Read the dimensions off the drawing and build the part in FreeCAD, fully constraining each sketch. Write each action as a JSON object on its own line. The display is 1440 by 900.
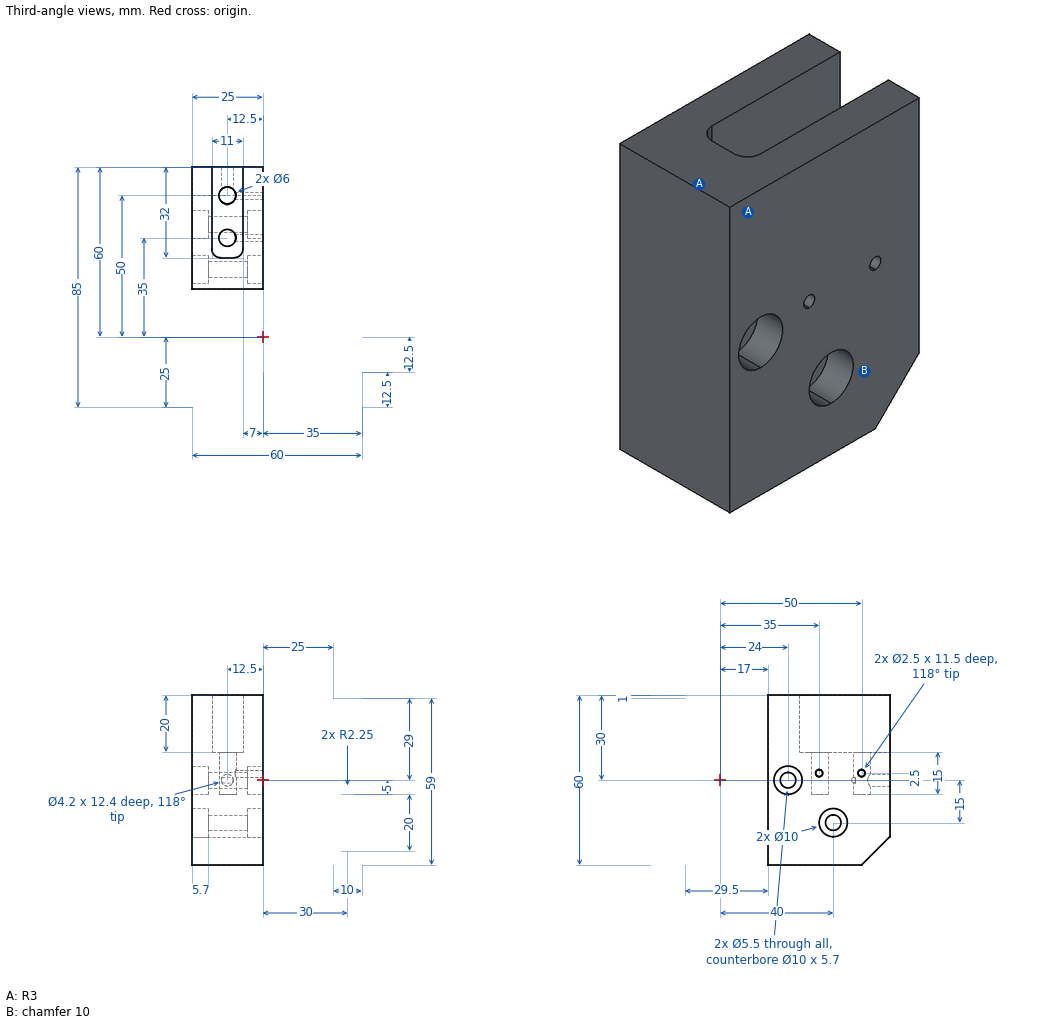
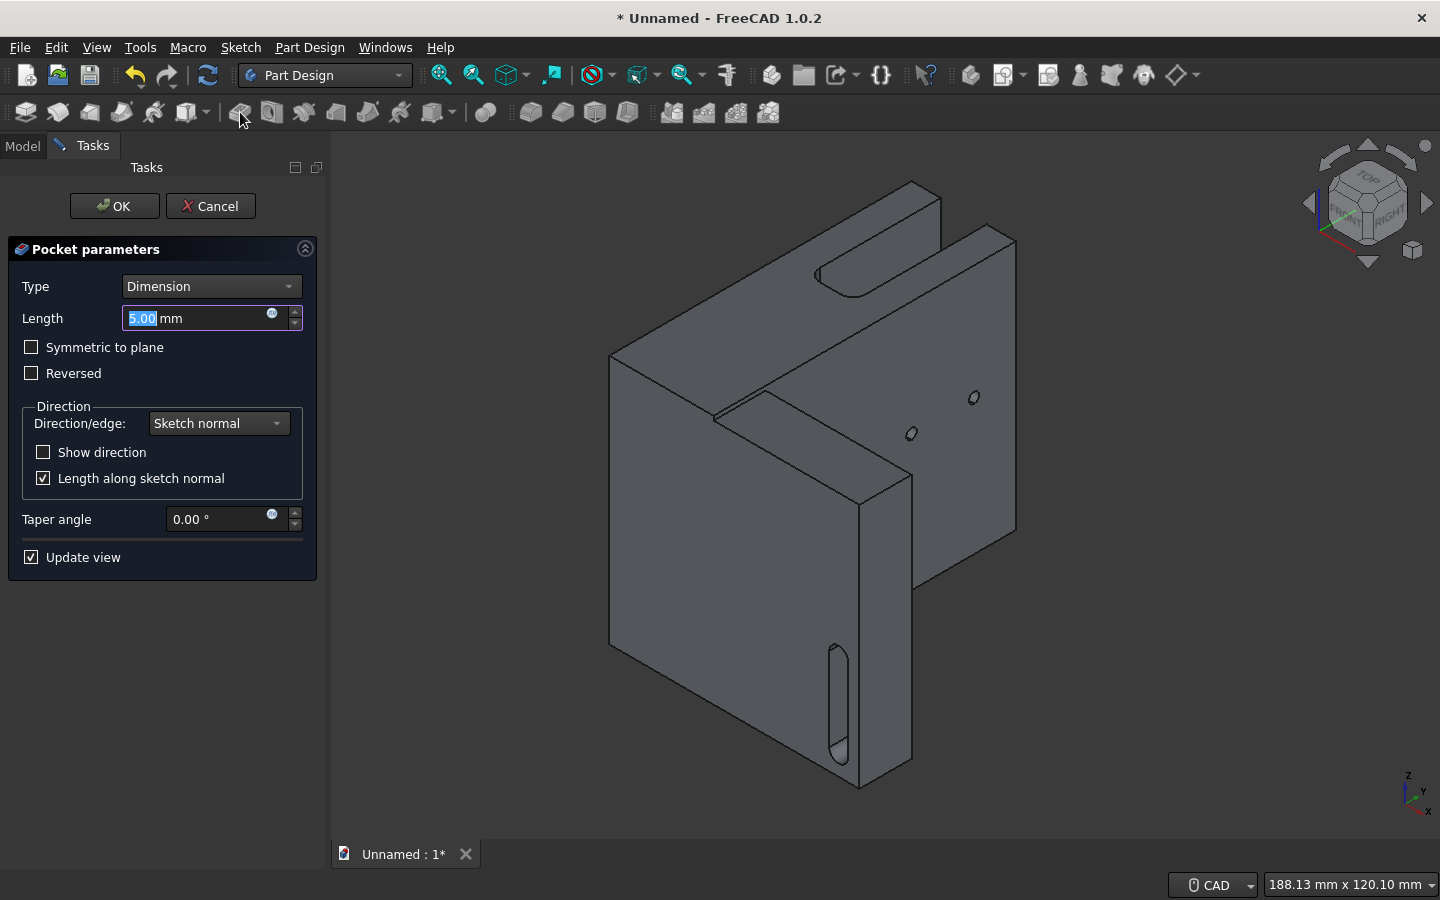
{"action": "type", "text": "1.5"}
{"action": "key", "text": "Tab"}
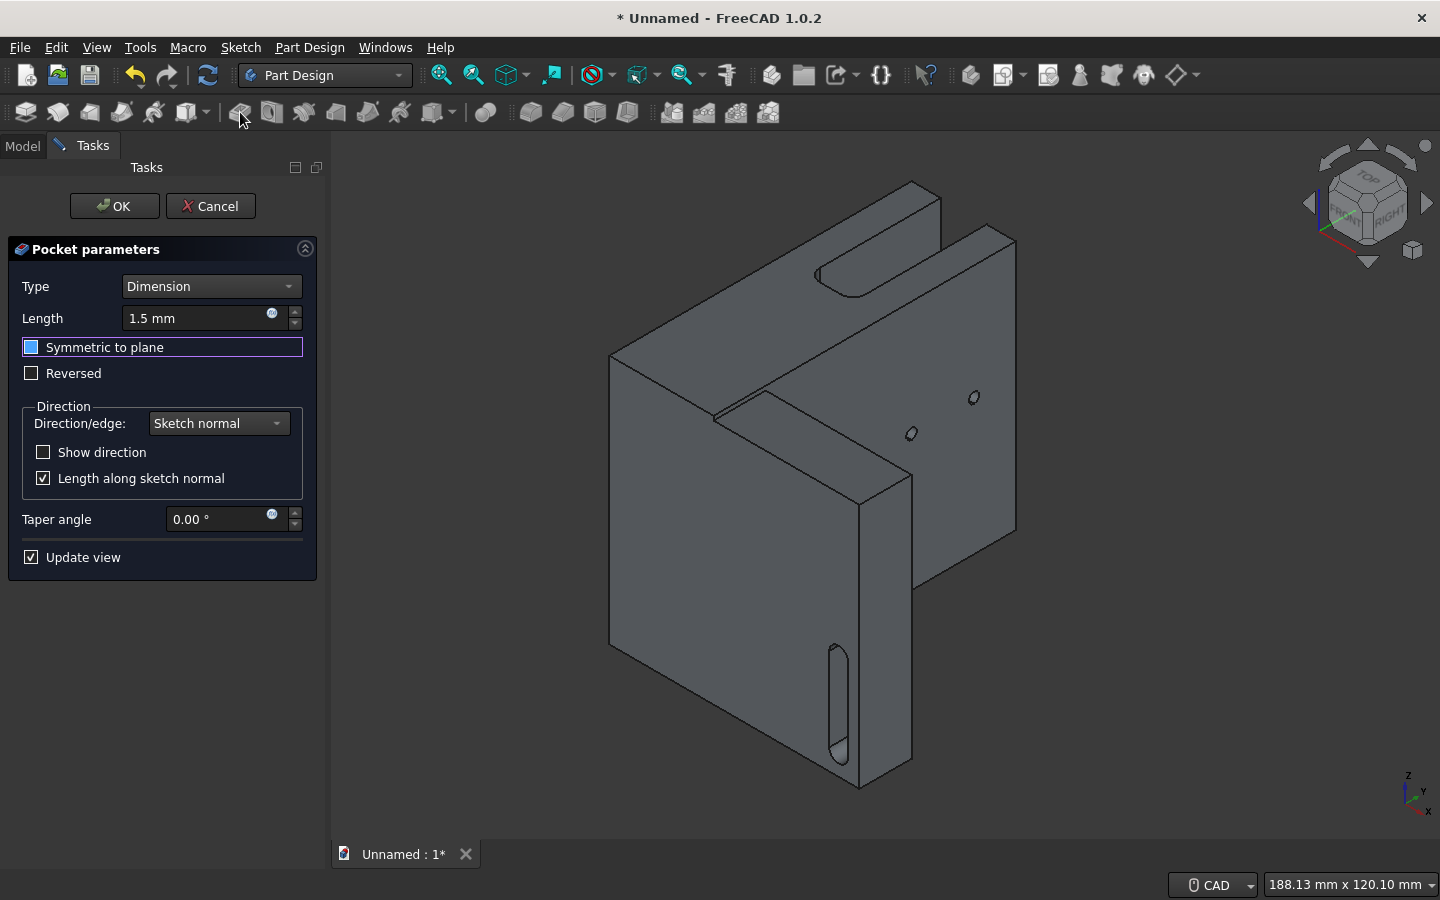
{"action": "left_click", "coordinate": [30, 373]}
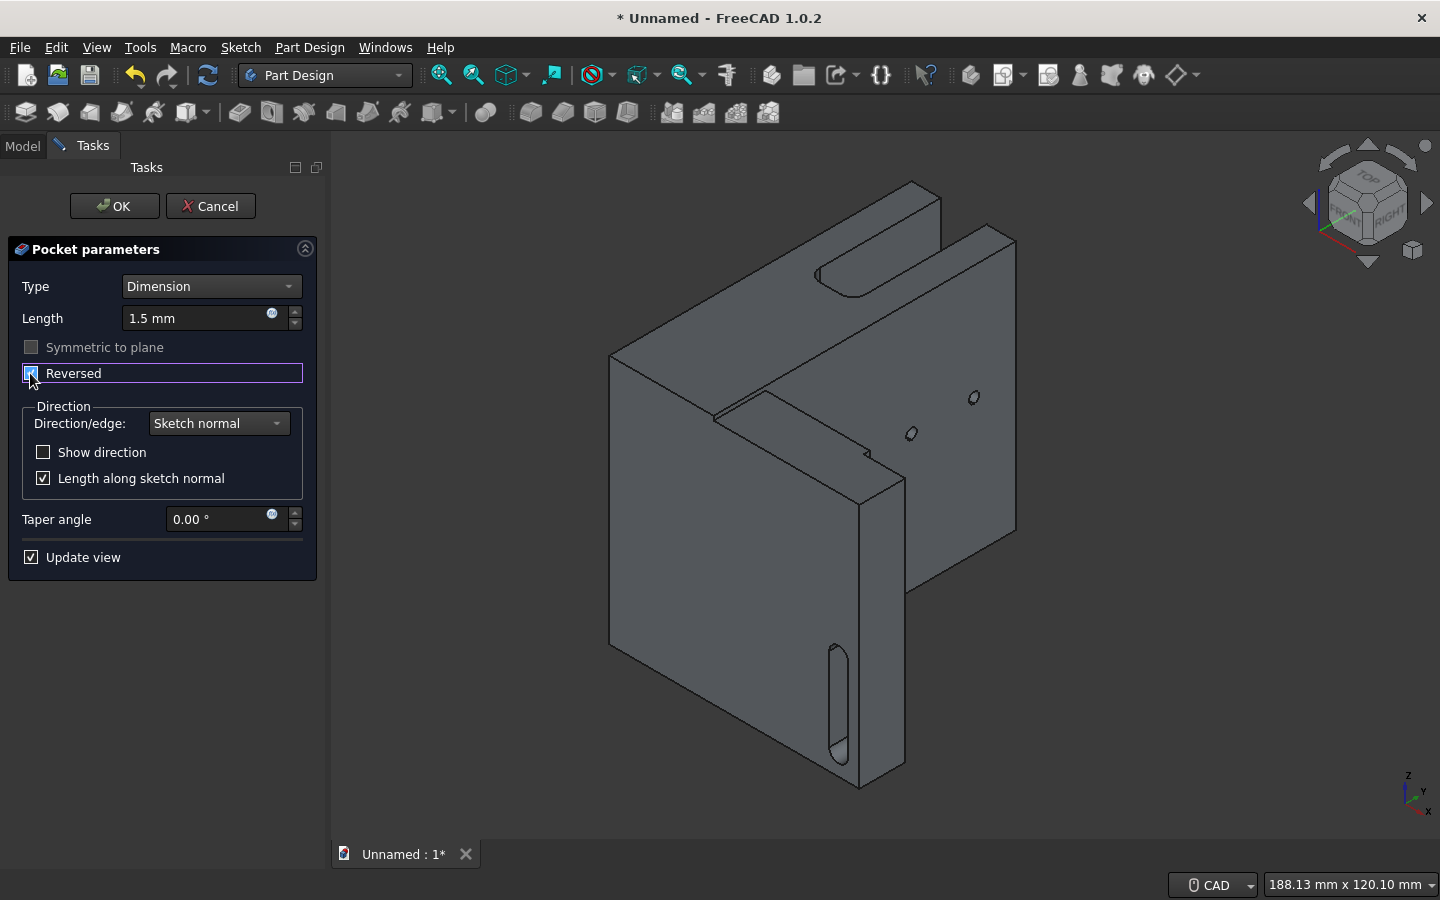
{"action": "left_click", "coordinate": [115, 206]}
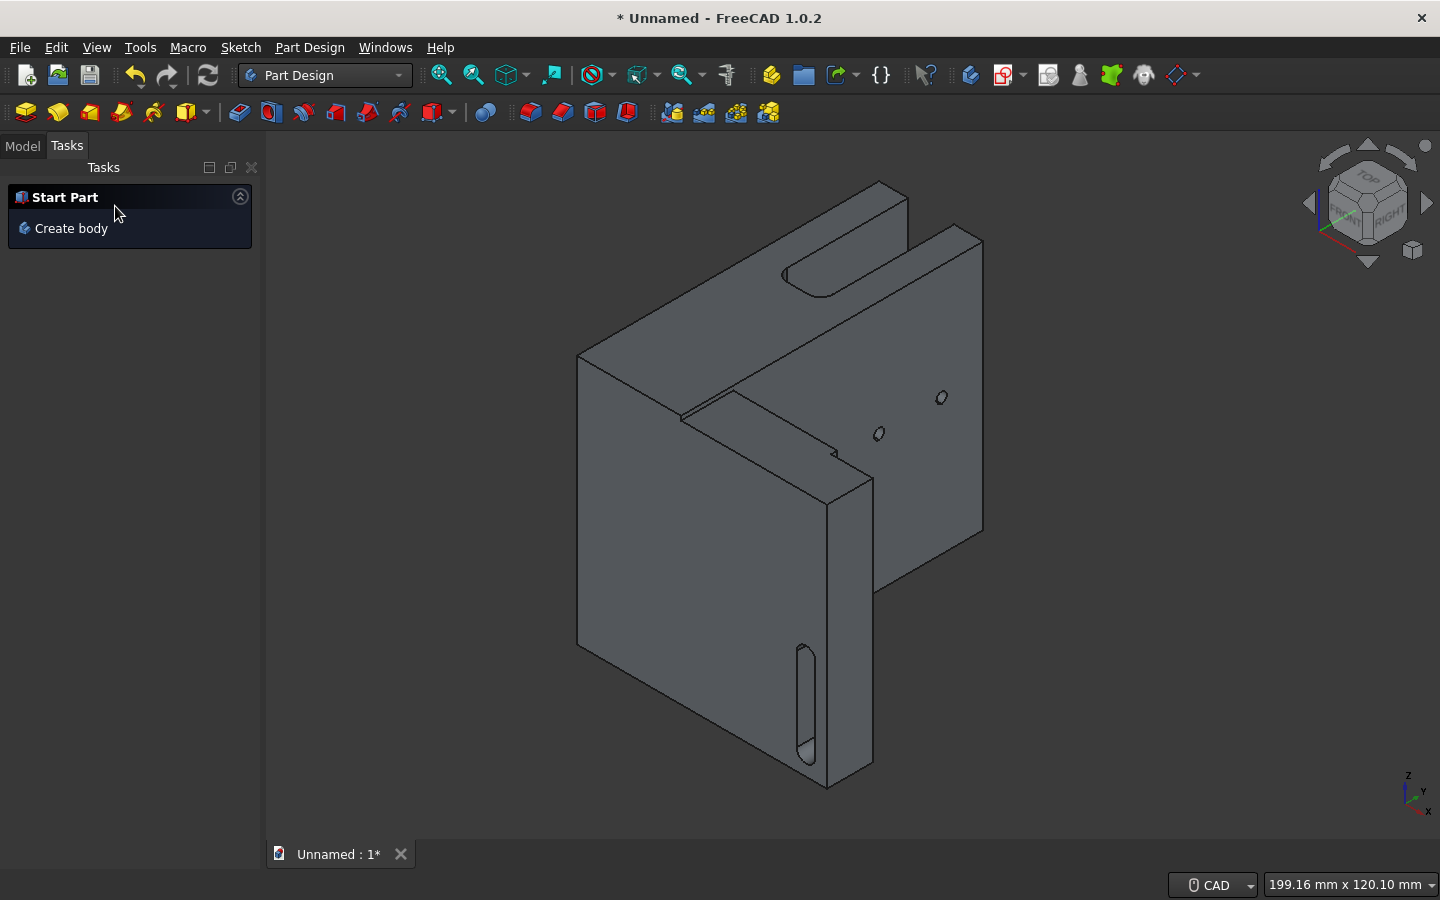
{"action": "key", "text": "2"}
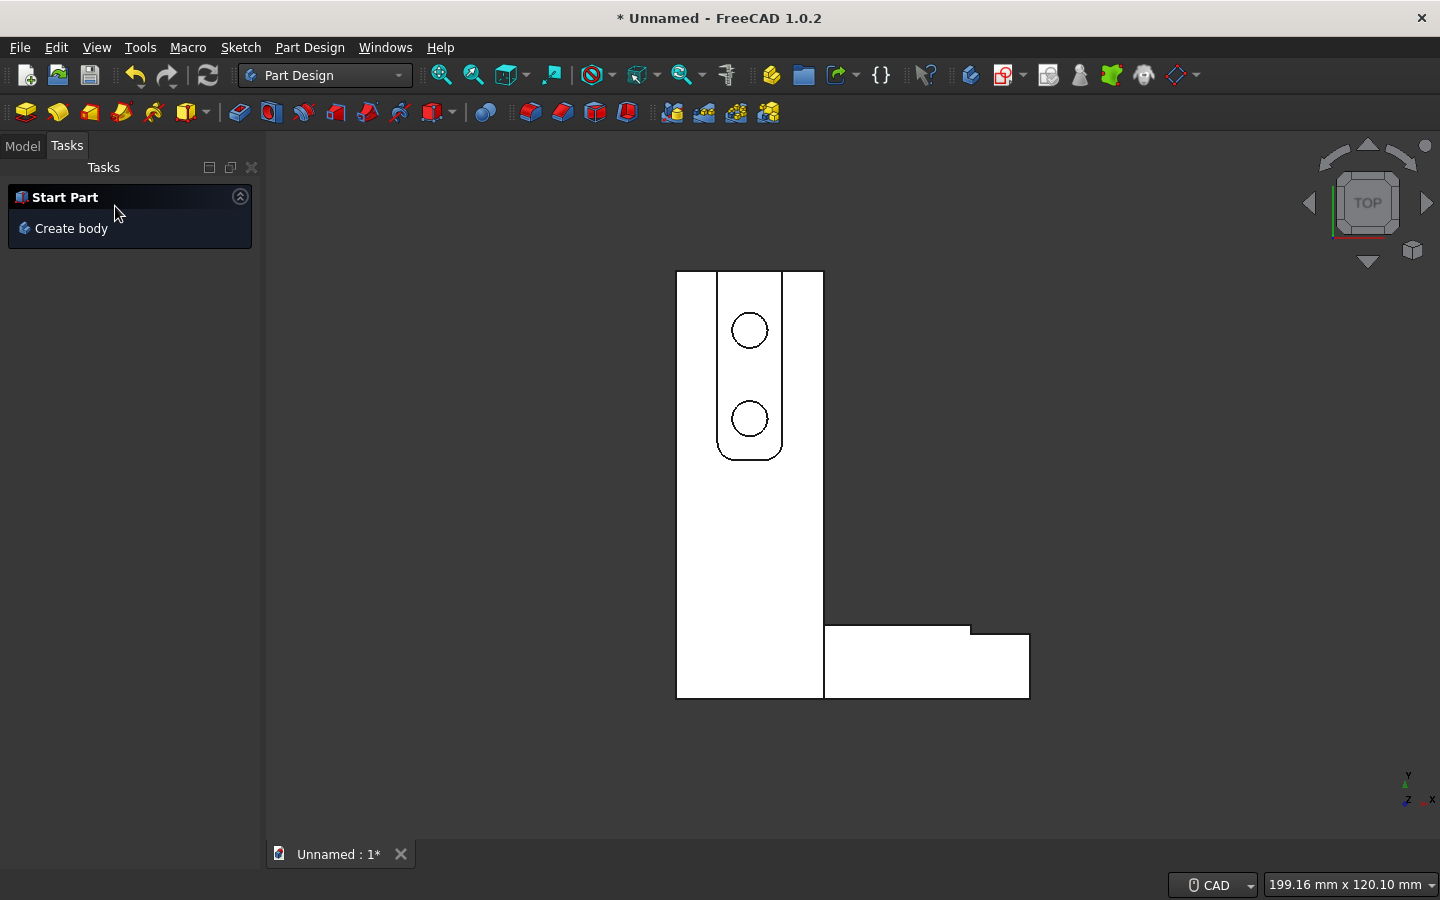
{"action": "key", "text": "0"}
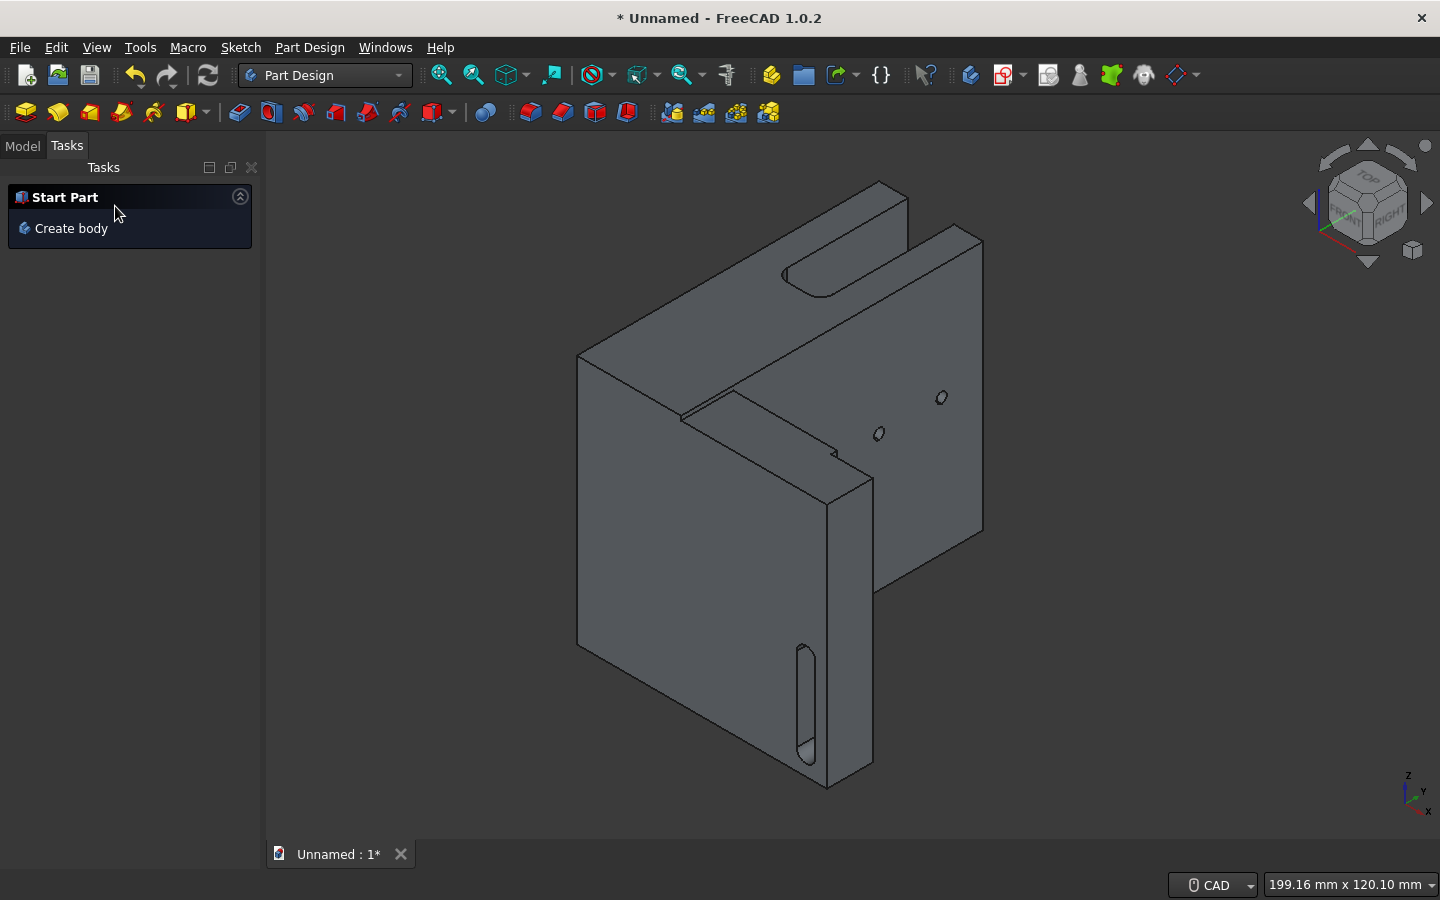
{"action": "key", "text": "1"}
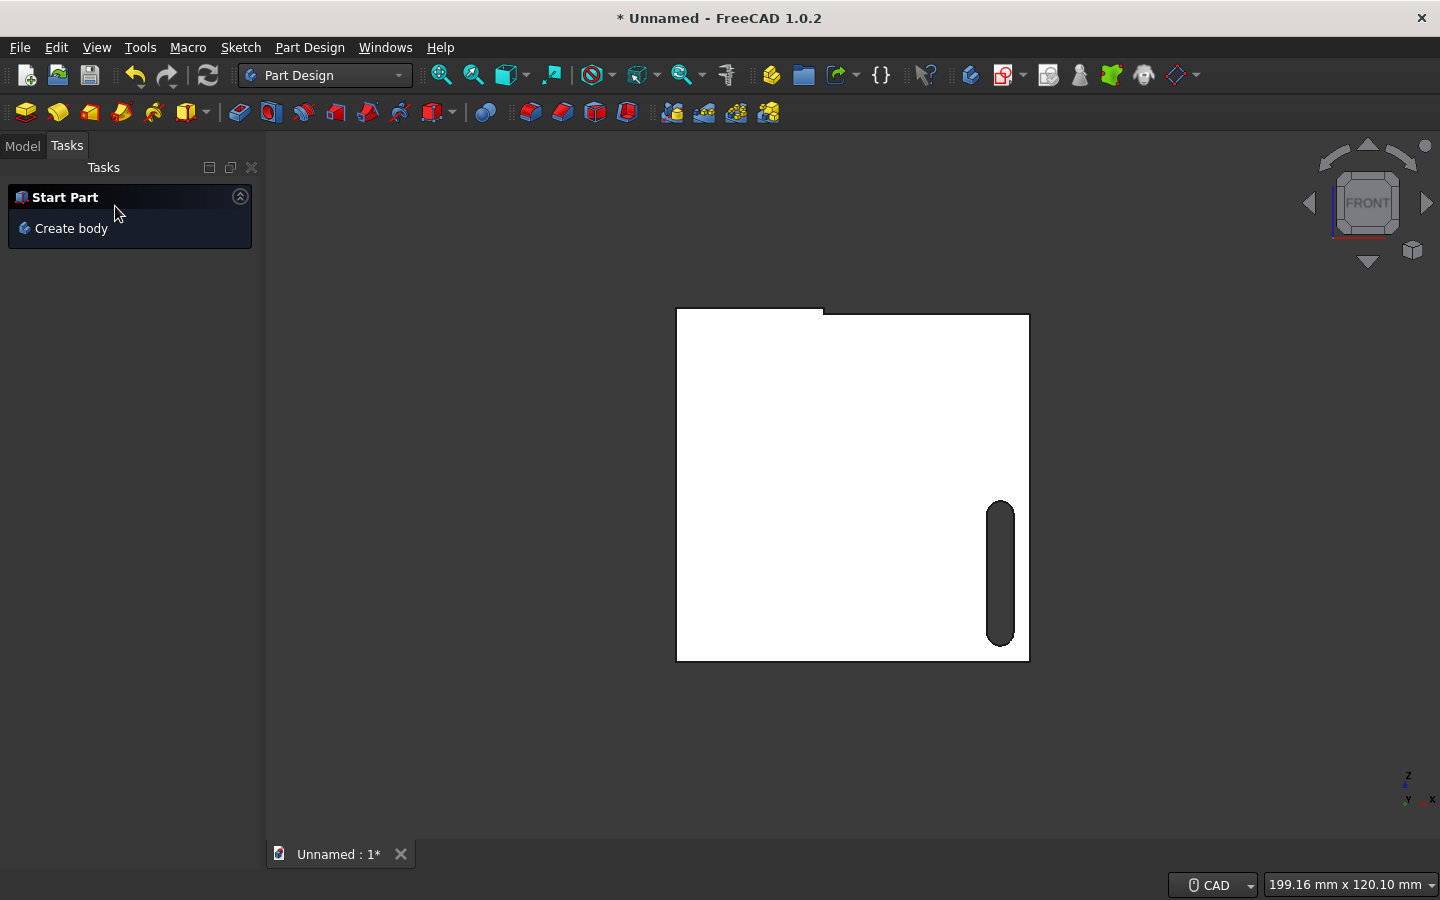
{"action": "key", "text": "3"}